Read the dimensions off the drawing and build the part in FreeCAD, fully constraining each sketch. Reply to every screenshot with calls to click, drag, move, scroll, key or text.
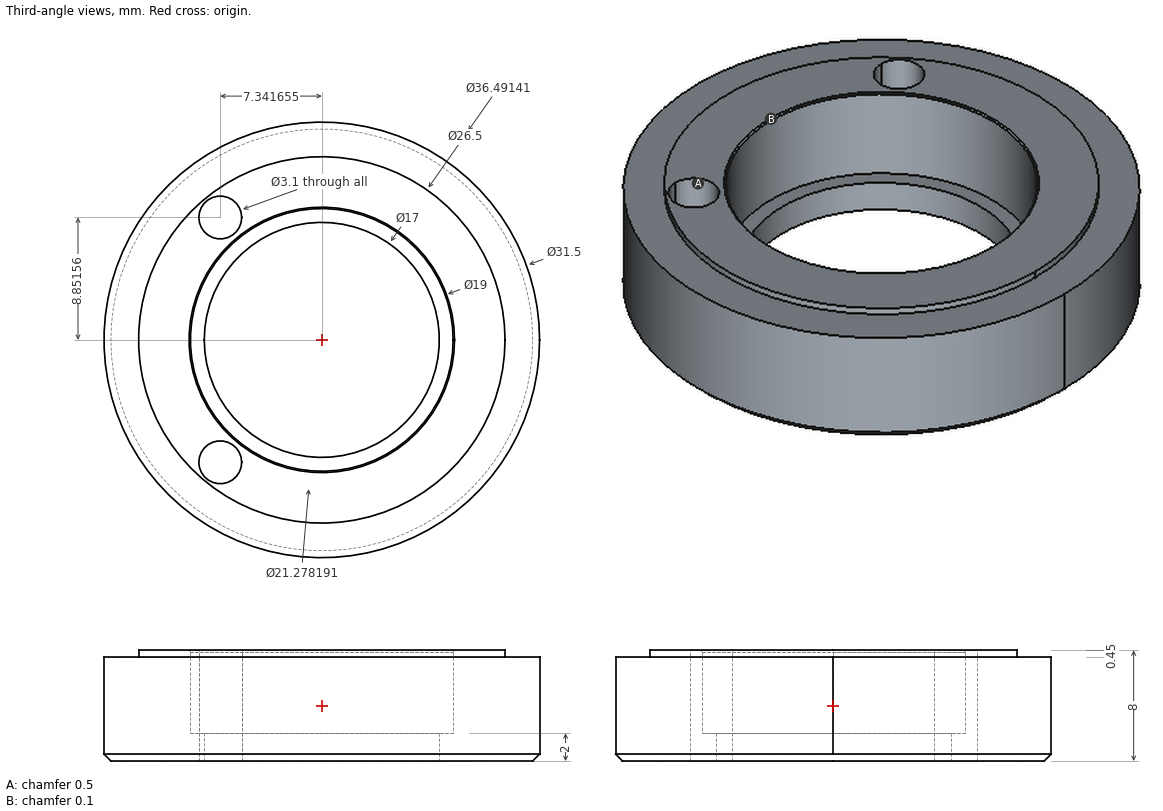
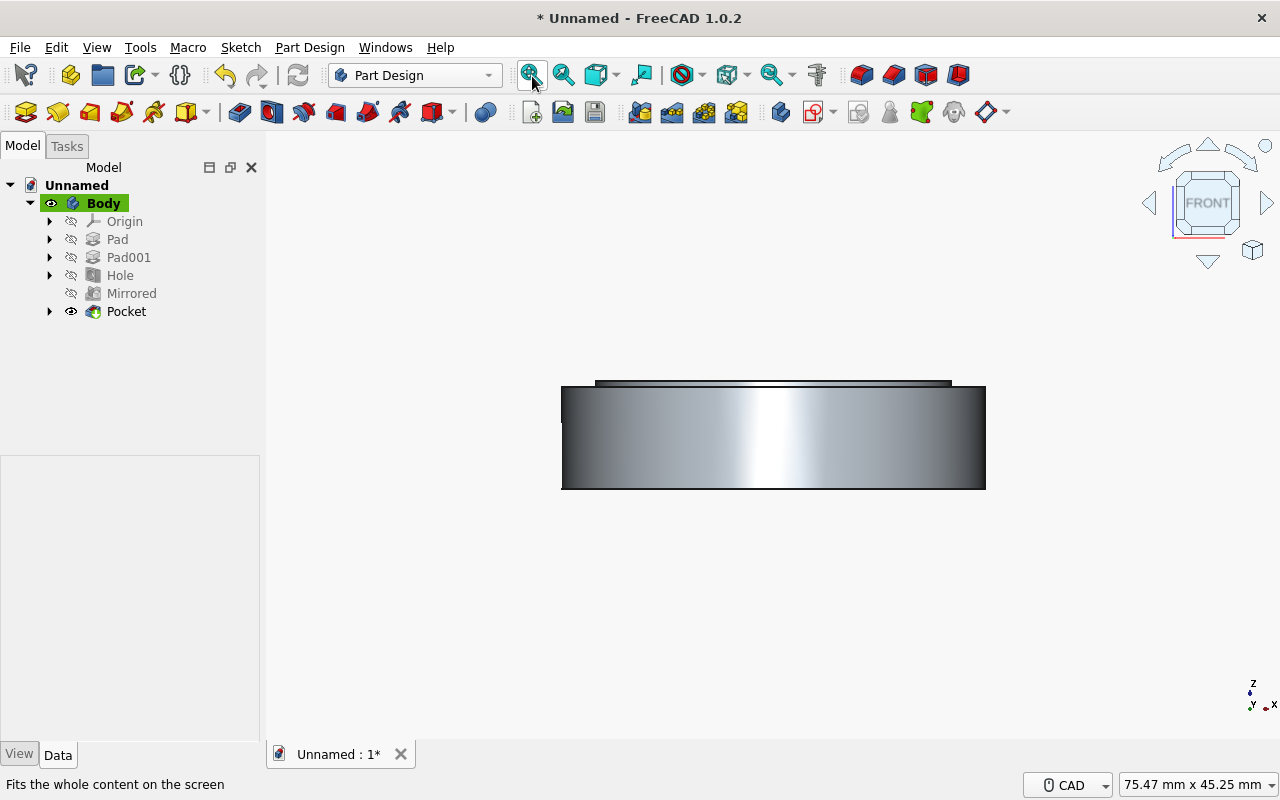
click(708, 488)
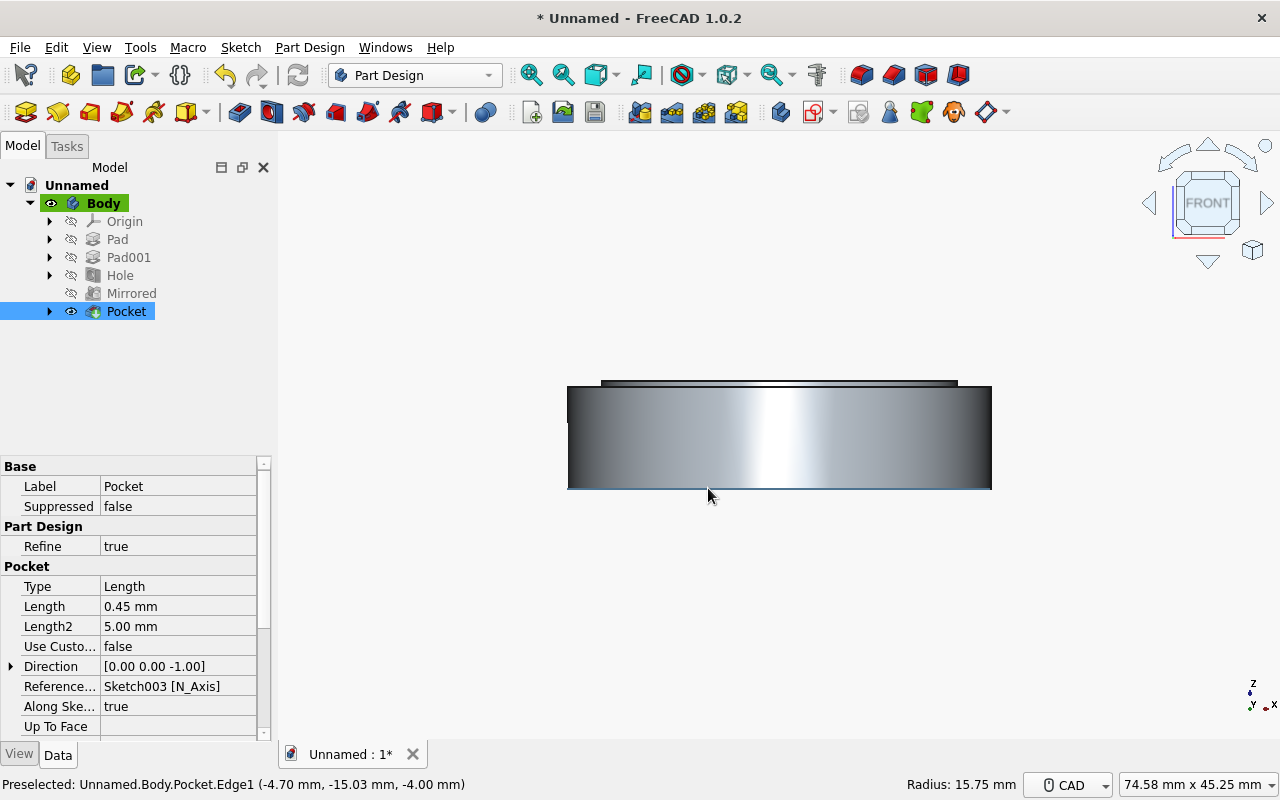
click(894, 76)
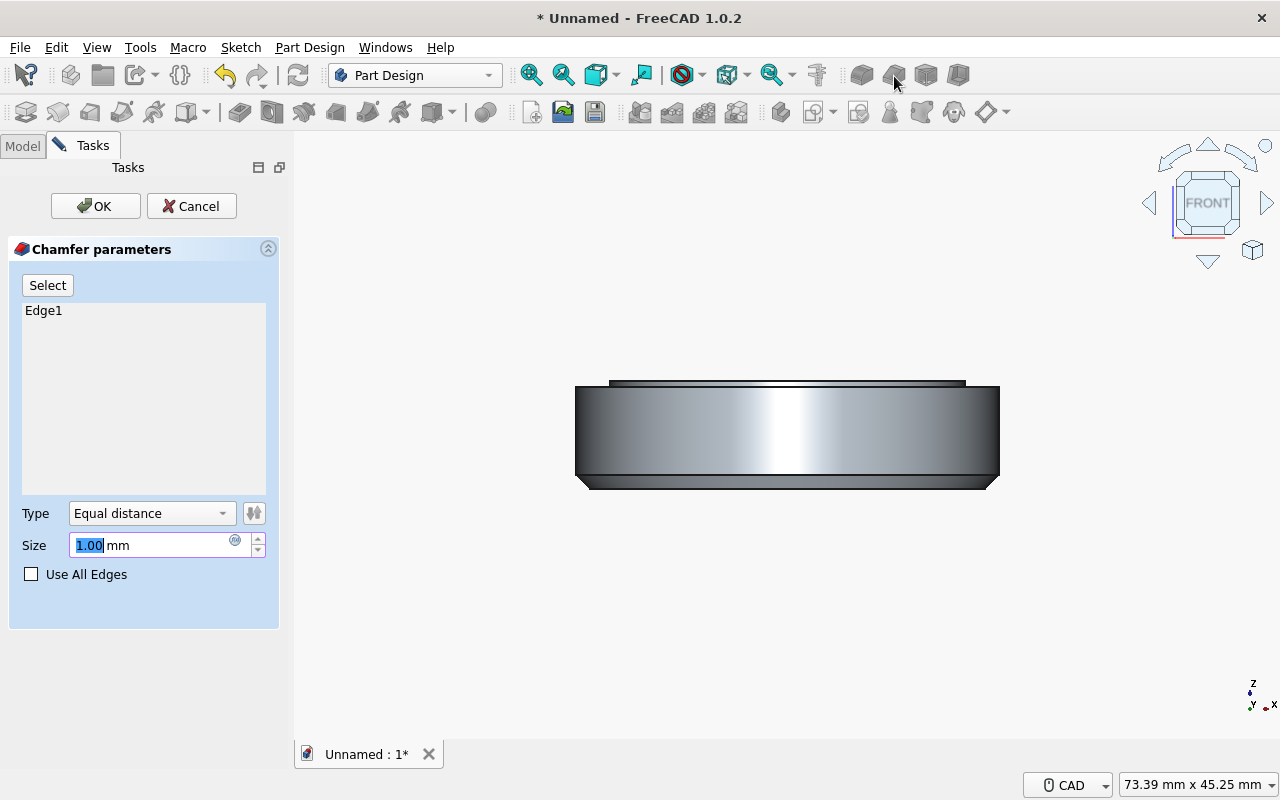
text(0.5)
key(Tab)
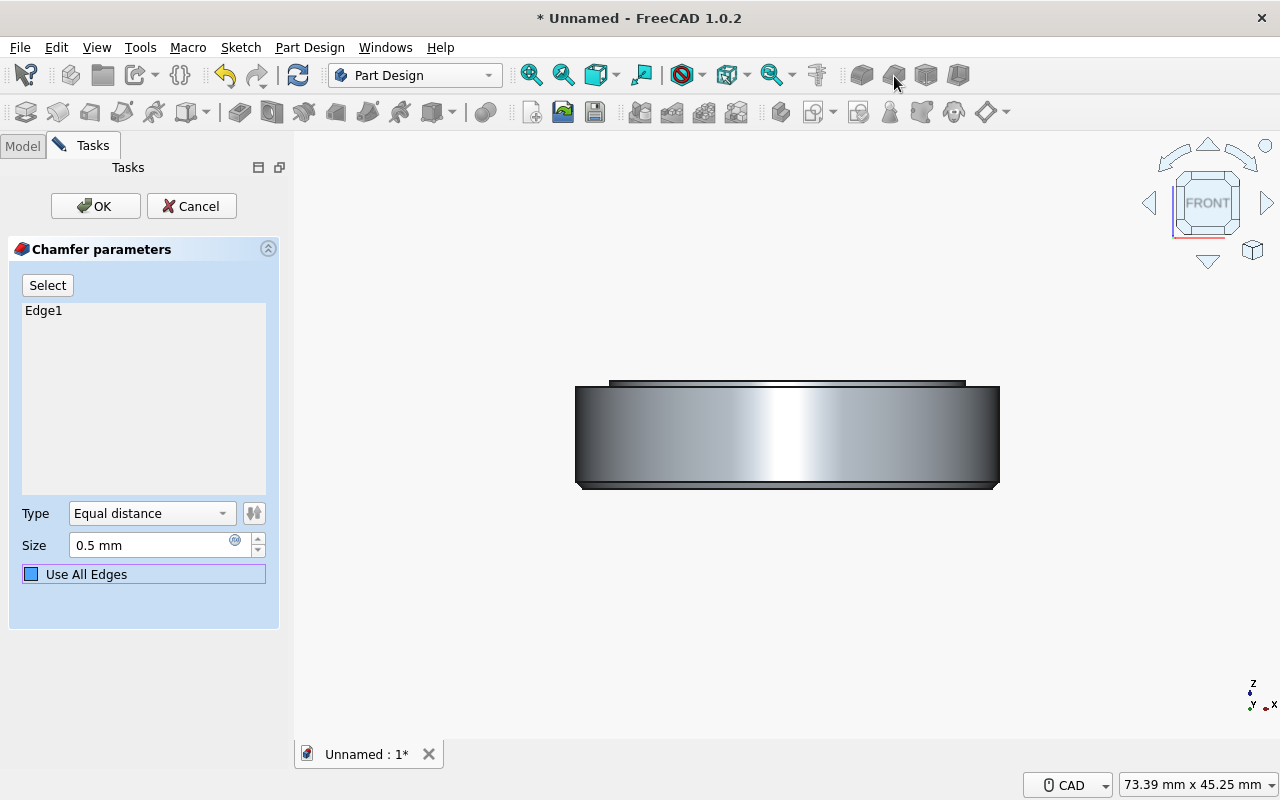
click(96, 206)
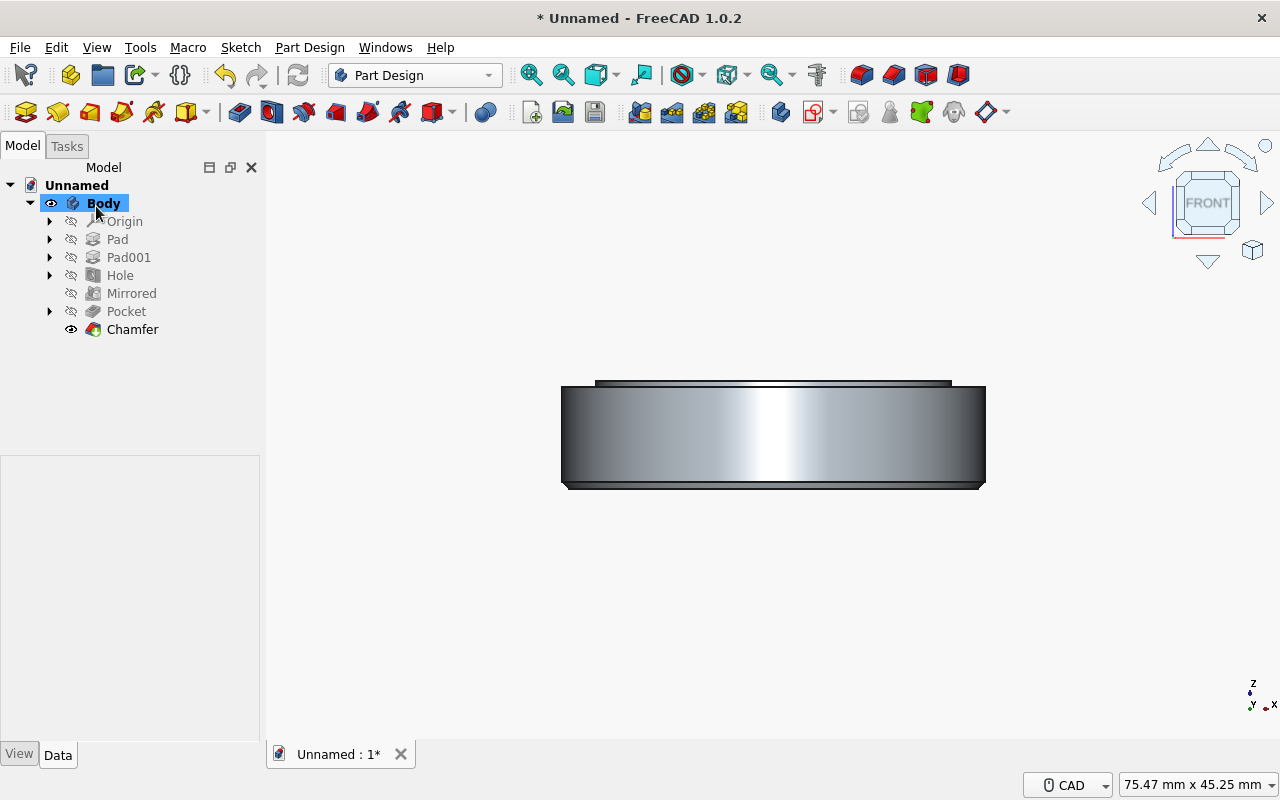
click(532, 76)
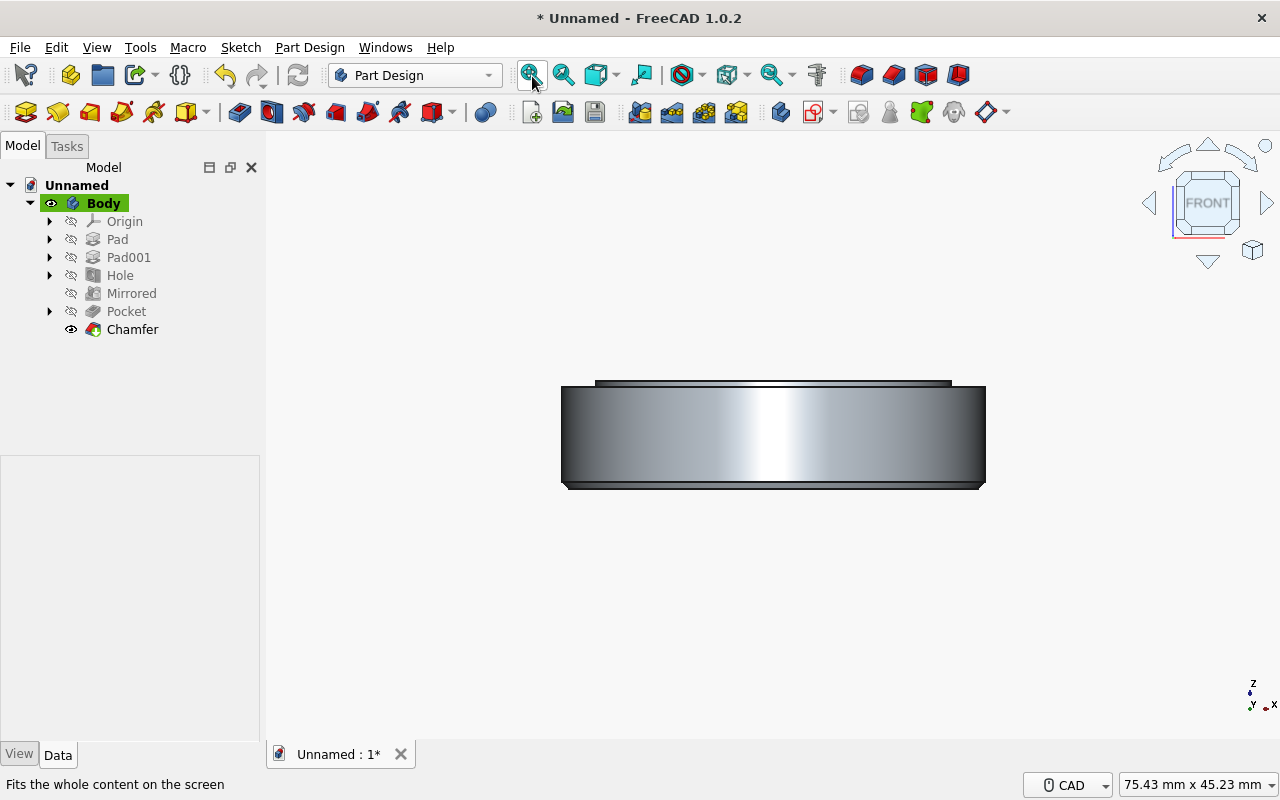
key(0)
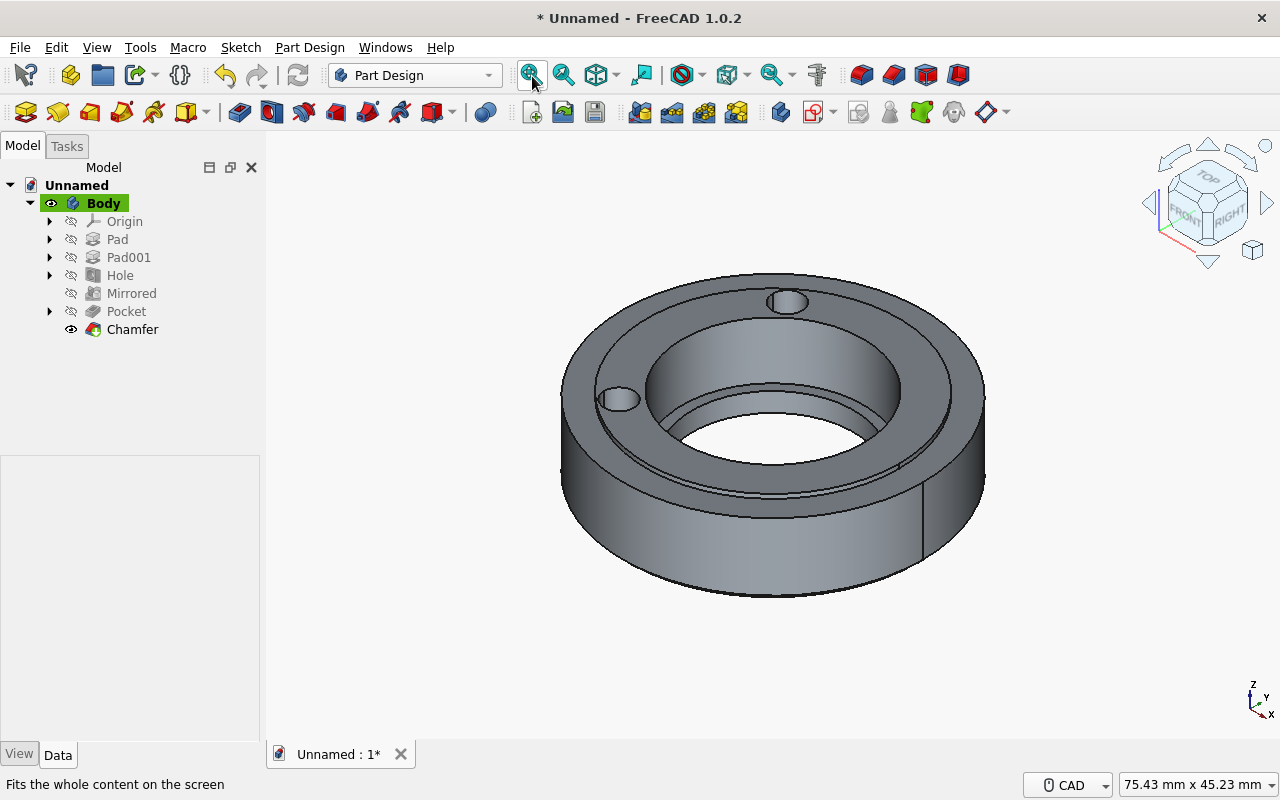
click(683, 338)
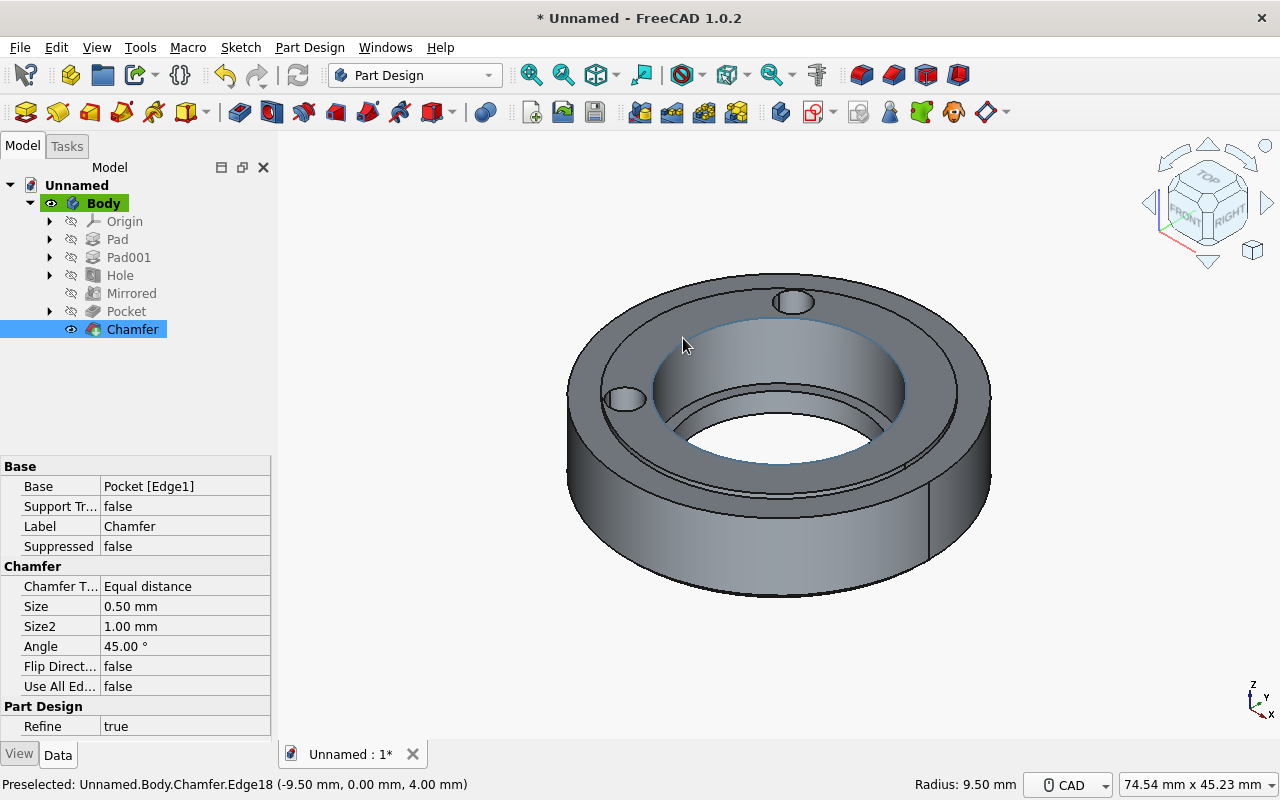
click(894, 76)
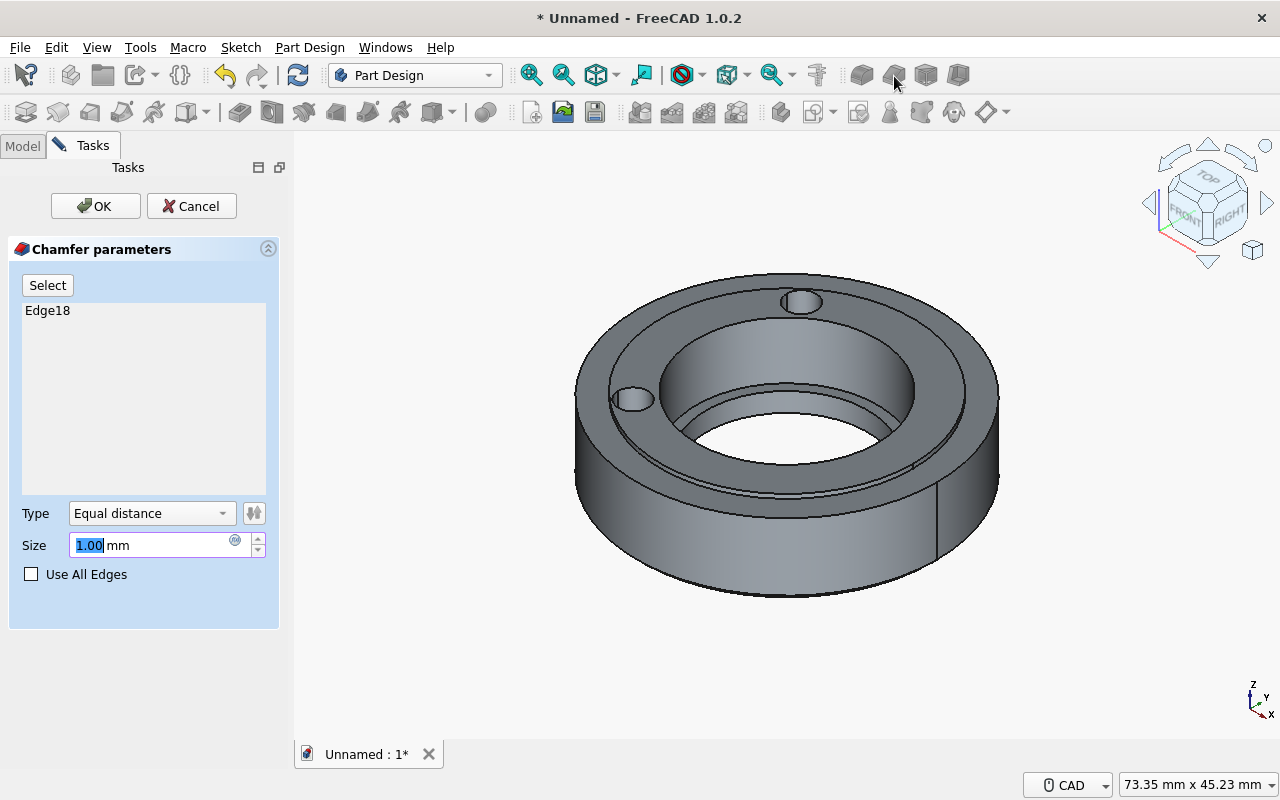
text(0.1)
key(Tab)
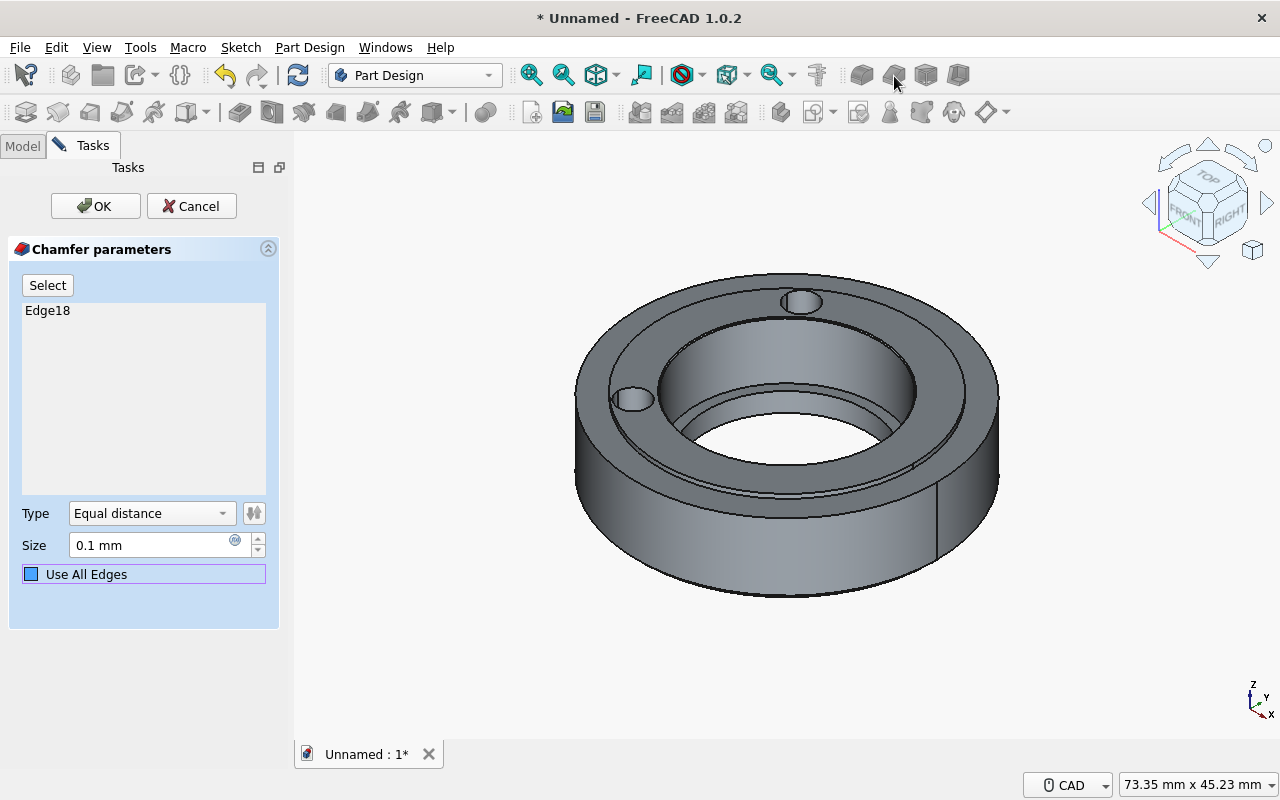
click(96, 206)